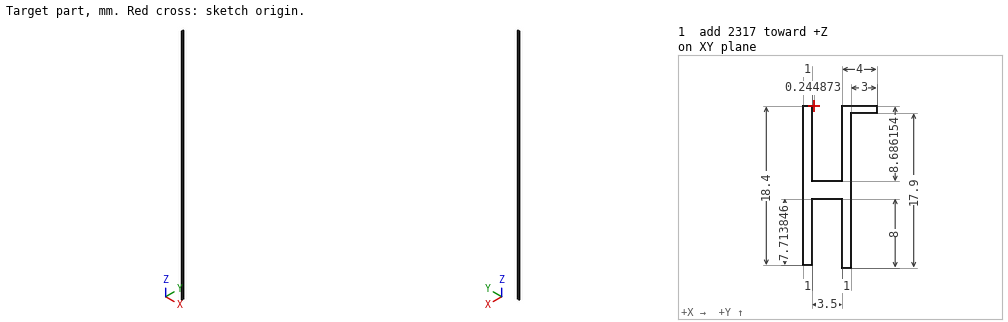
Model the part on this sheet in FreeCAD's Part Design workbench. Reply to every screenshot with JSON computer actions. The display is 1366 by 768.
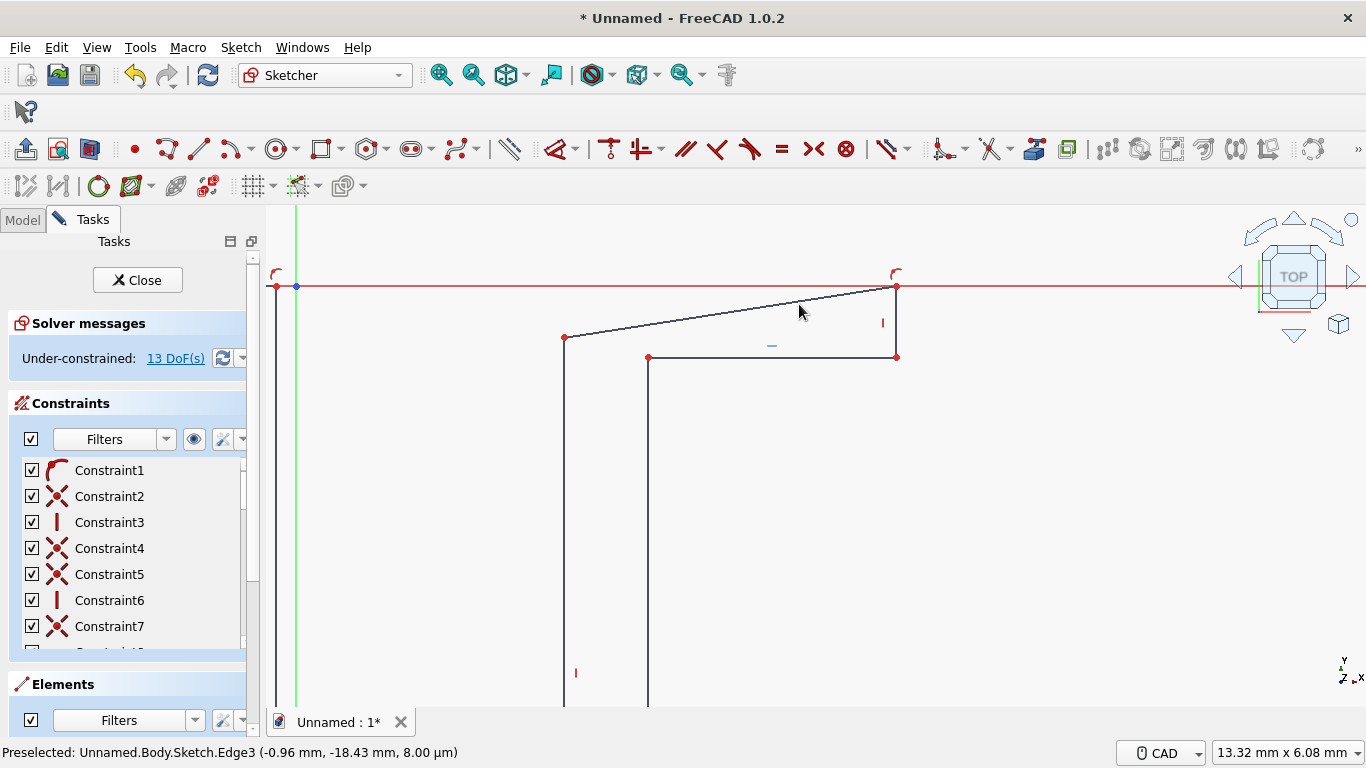
{"action": "left_click", "coordinate": [797, 302]}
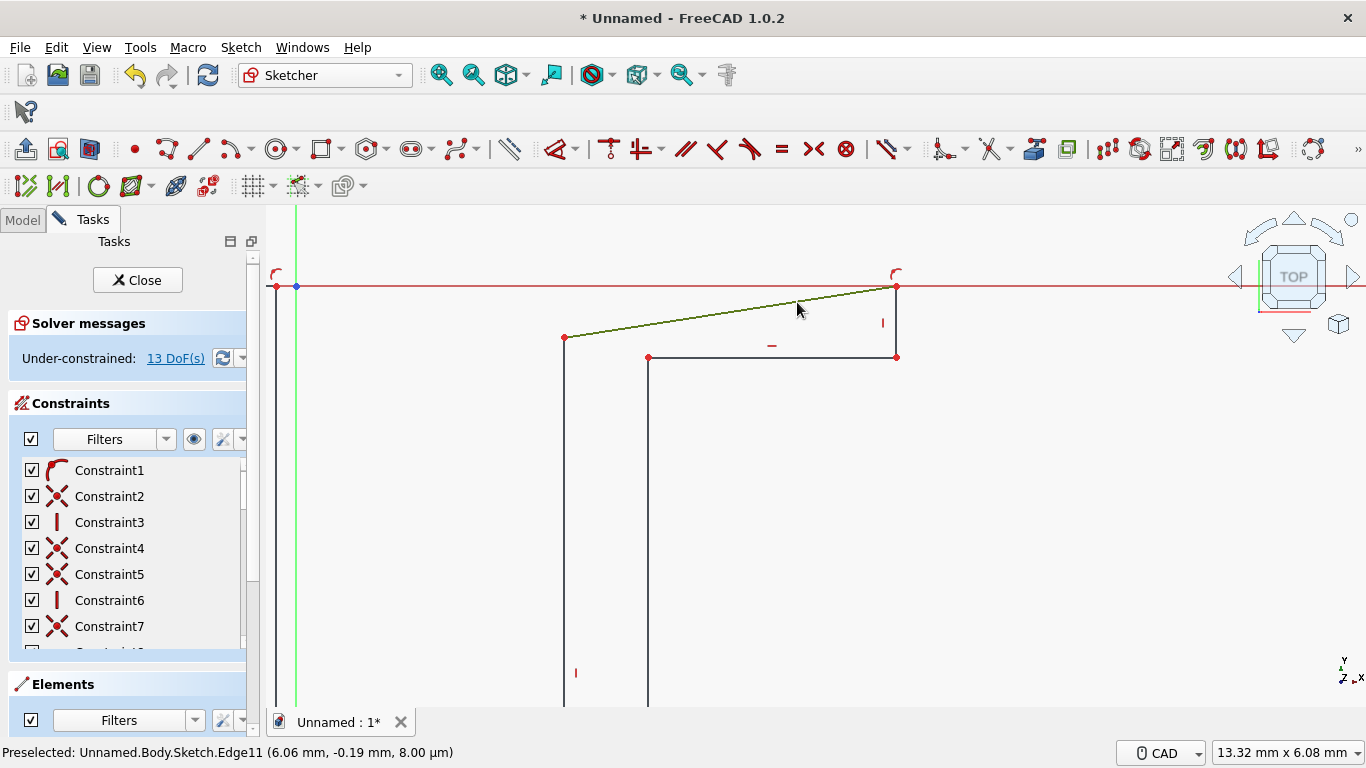
{"action": "key", "text": "h"}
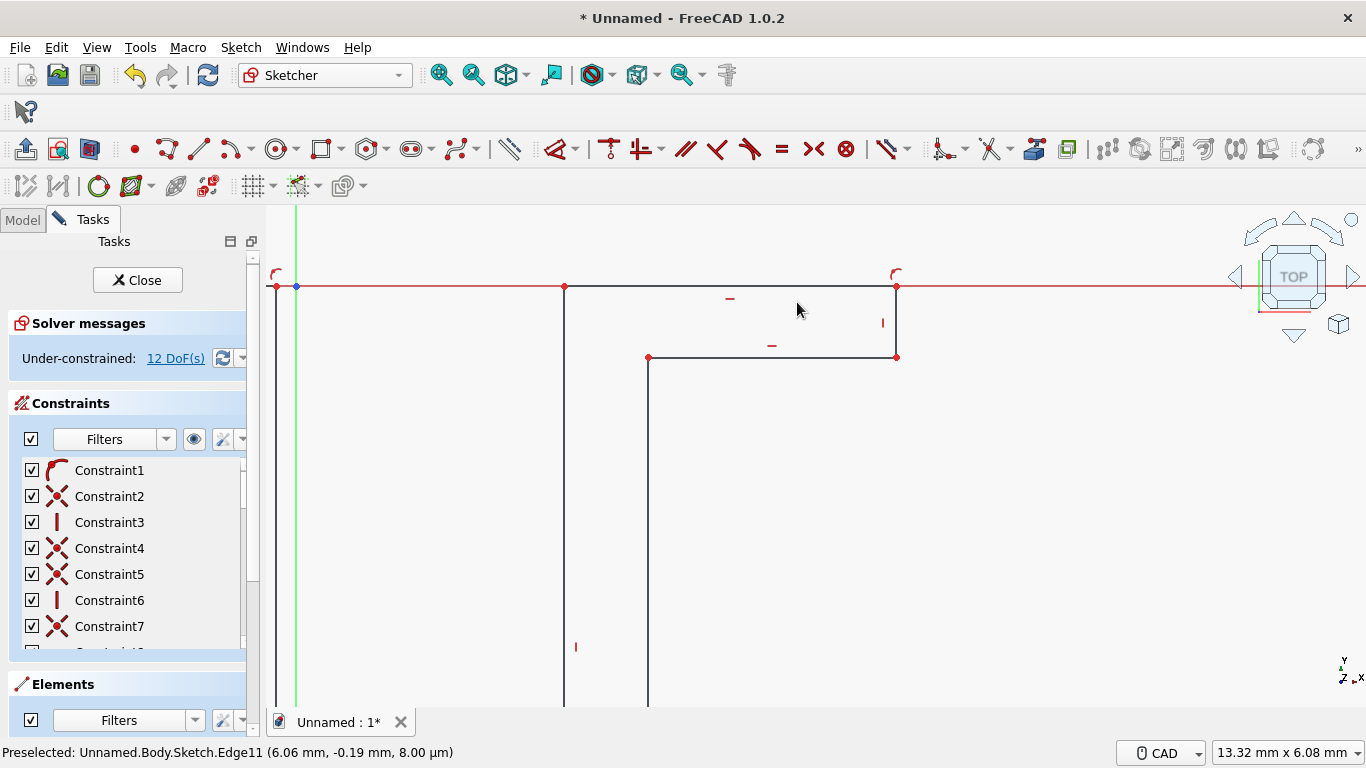
{"action": "scroll", "coordinate": [799, 304], "scroll_direction": "down", "scroll_amount": 8}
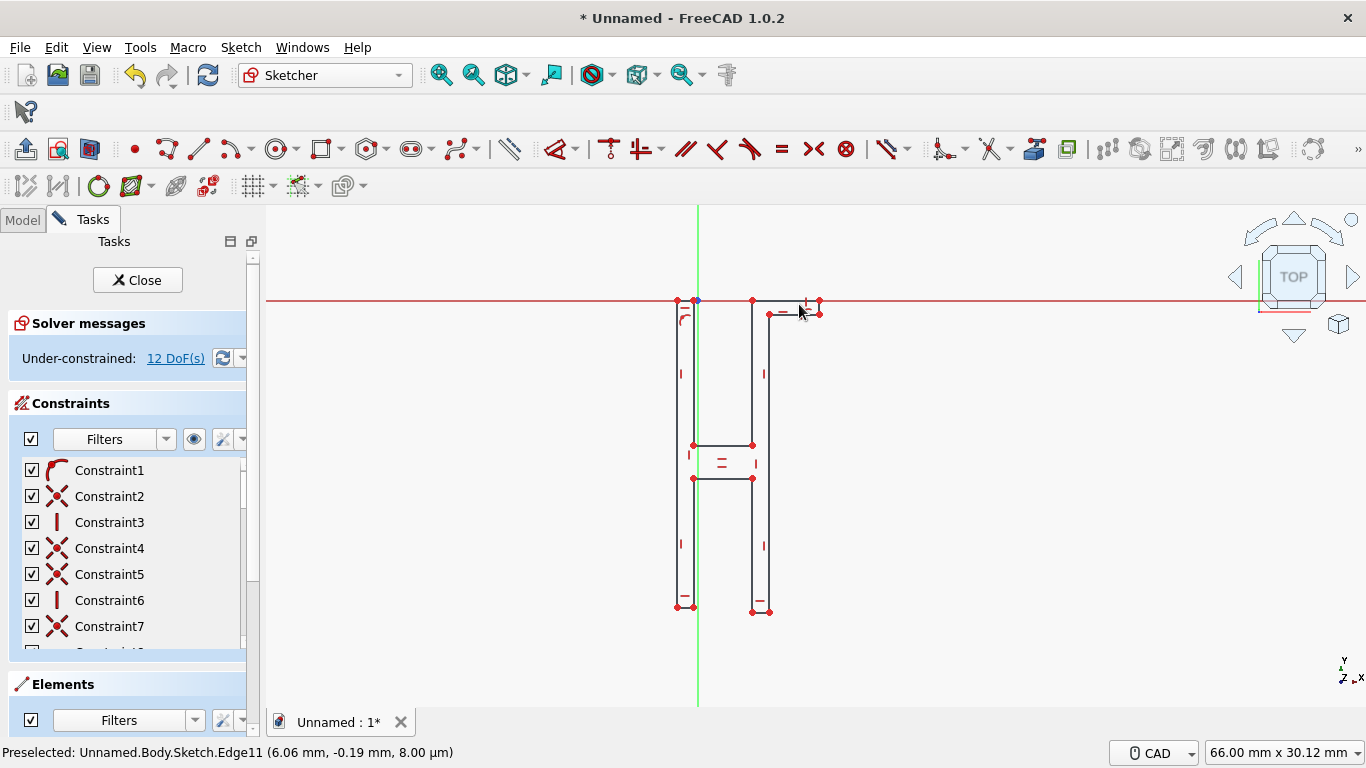
{"action": "scroll", "coordinate": [689, 301], "scroll_direction": "up", "scroll_amount": 6}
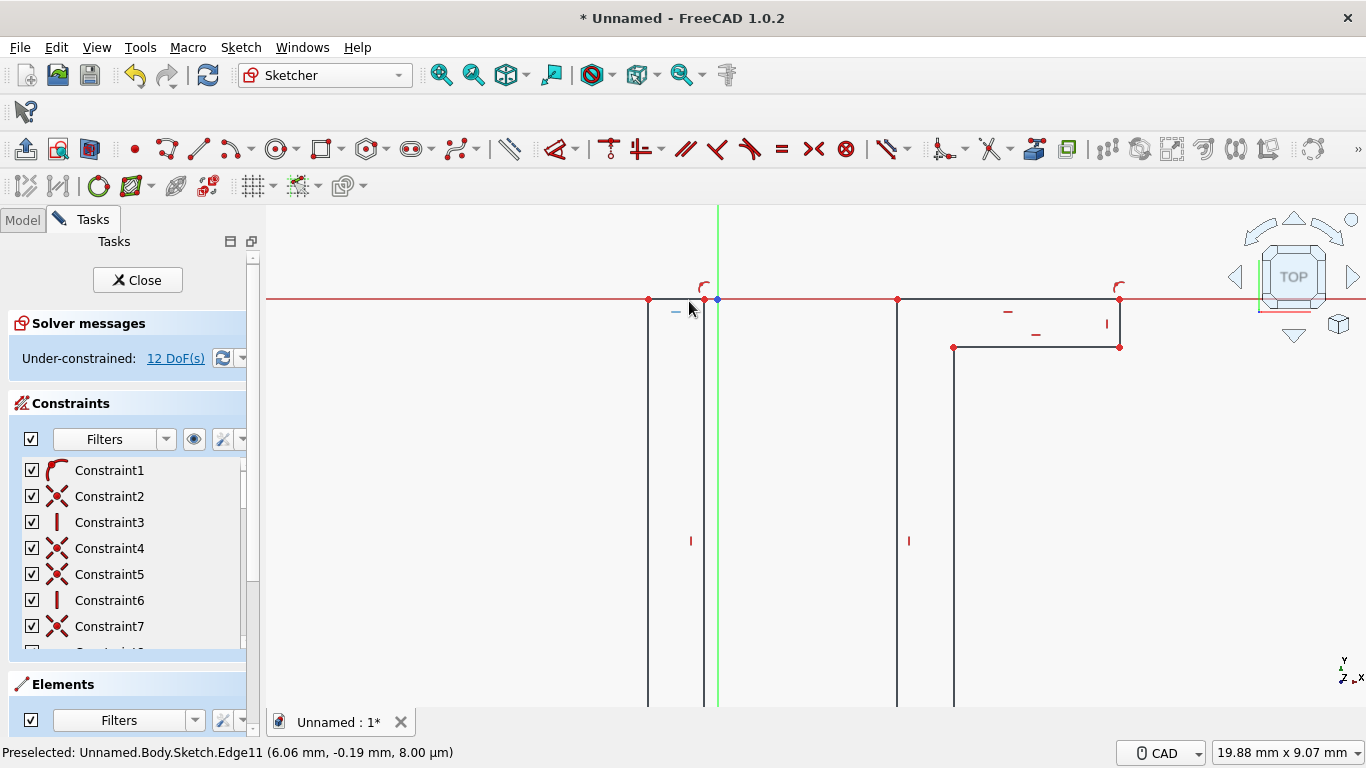
{"action": "left_click", "coordinate": [687, 299]}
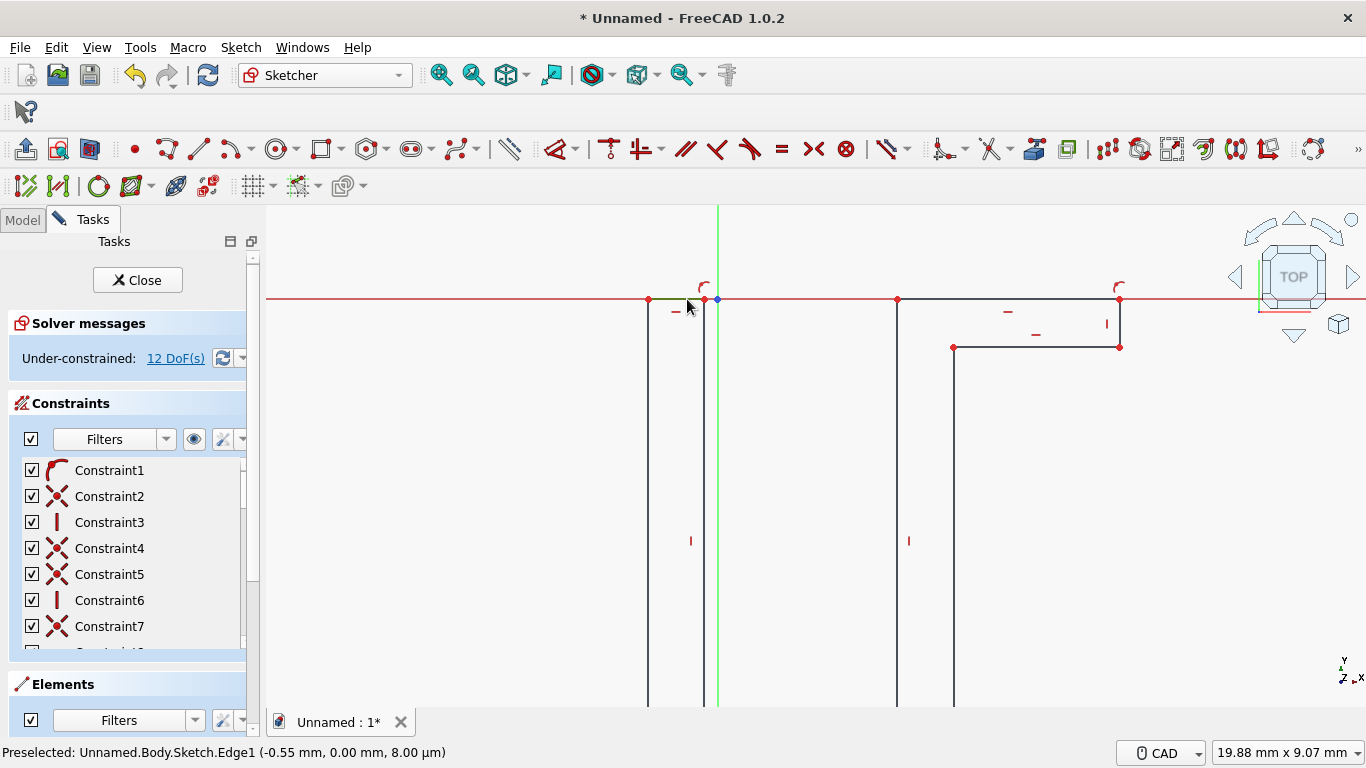
{"action": "key", "text": "l"}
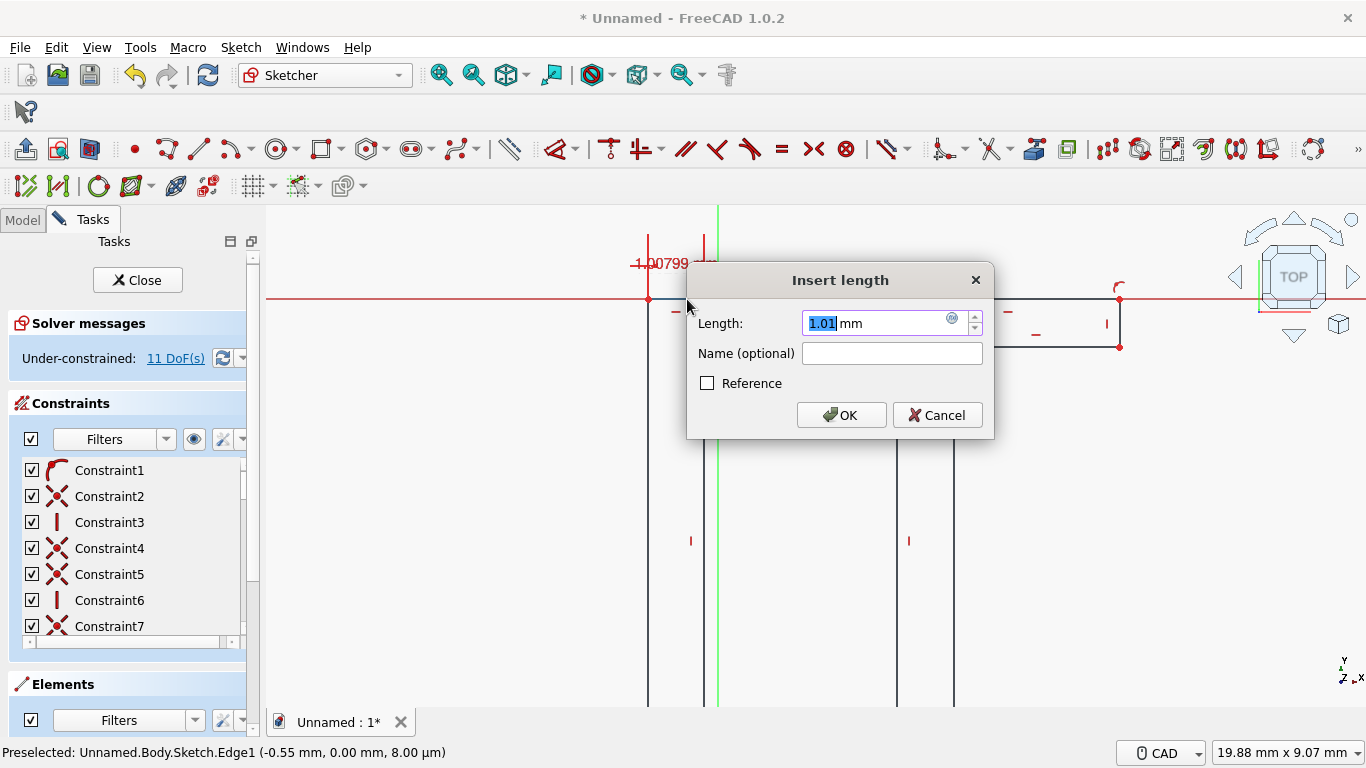
{"action": "type", "text": "1"}
{"action": "key", "text": "Return"}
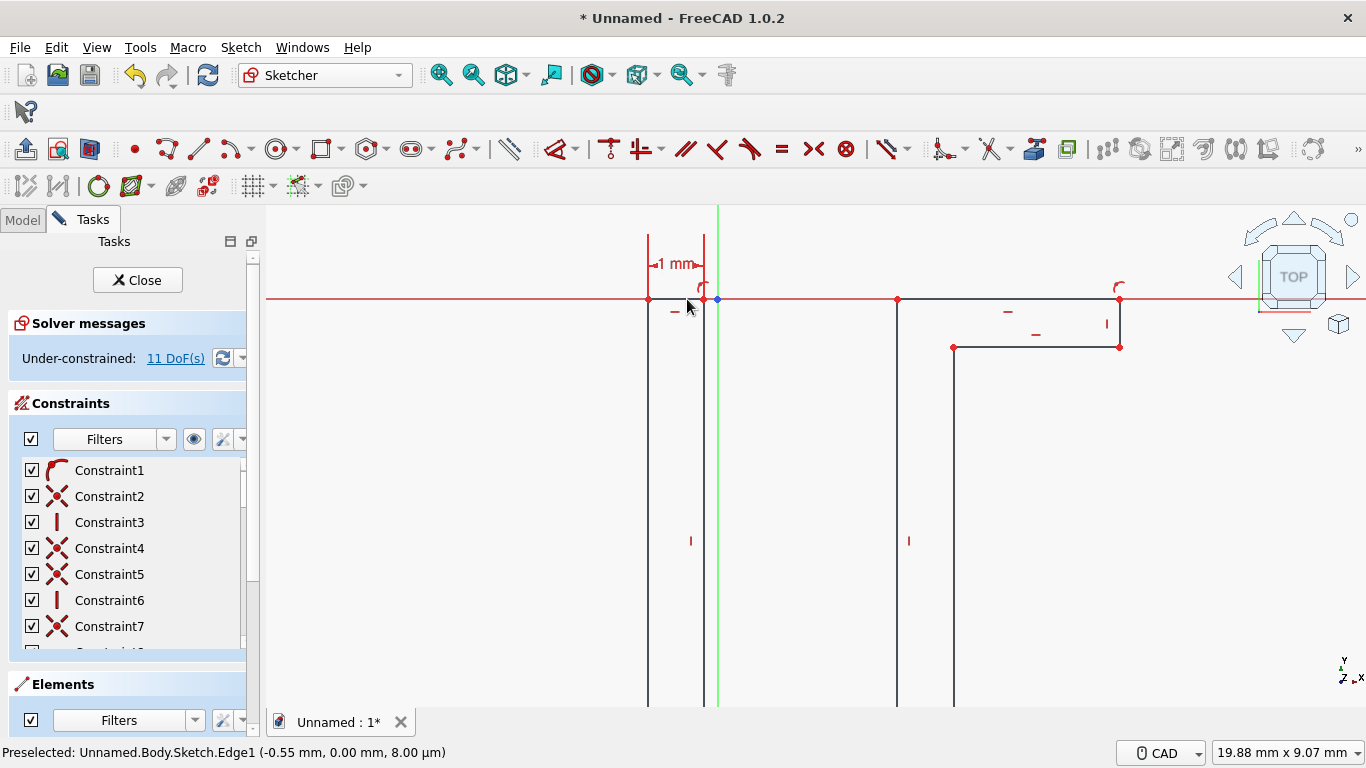
{"action": "scroll", "coordinate": [689, 301], "scroll_direction": "down", "scroll_amount": 6}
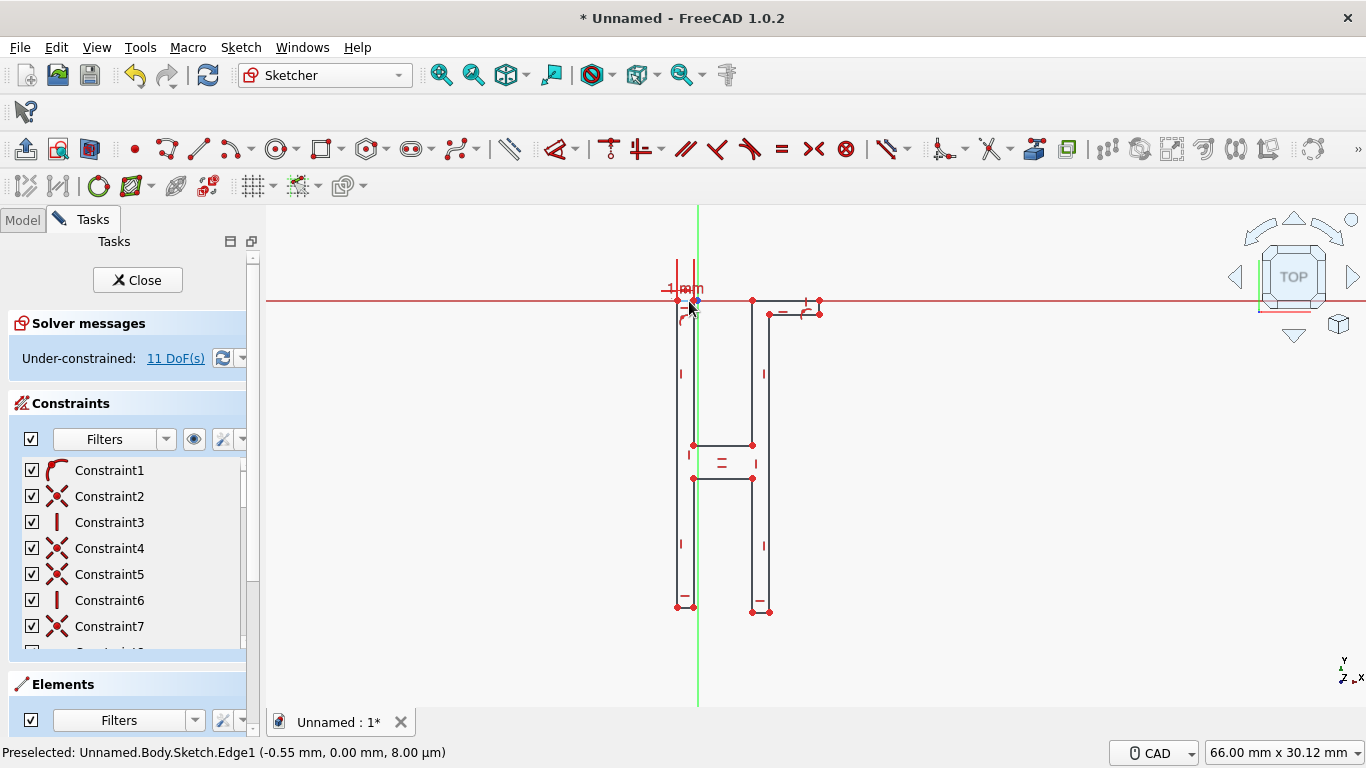
{"action": "scroll", "coordinate": [682, 608], "scroll_direction": "up", "scroll_amount": 6}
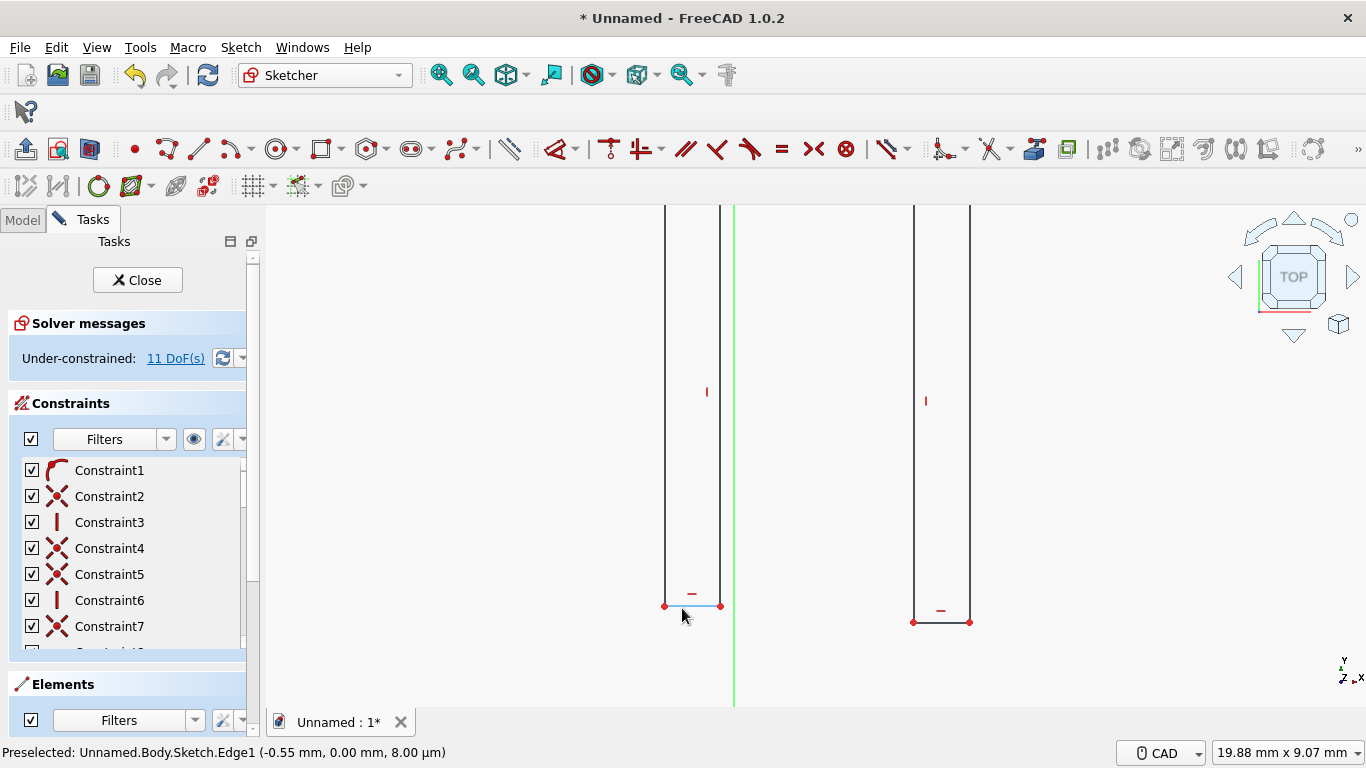
{"action": "left_click", "coordinate": [681, 606]}